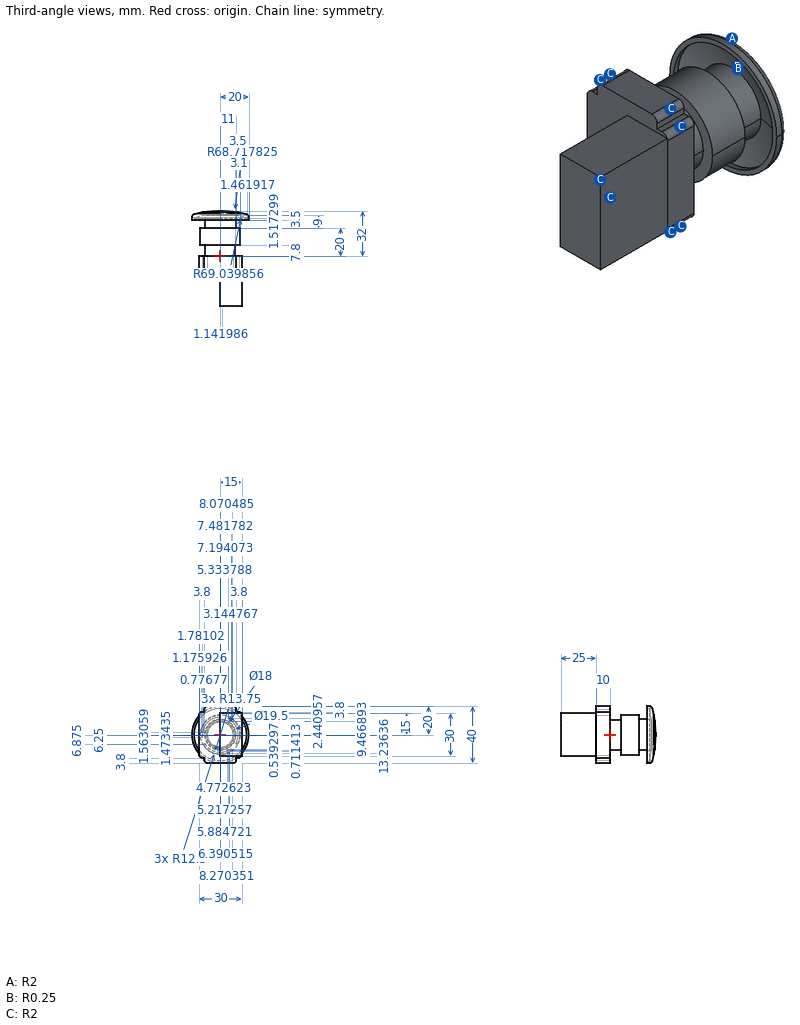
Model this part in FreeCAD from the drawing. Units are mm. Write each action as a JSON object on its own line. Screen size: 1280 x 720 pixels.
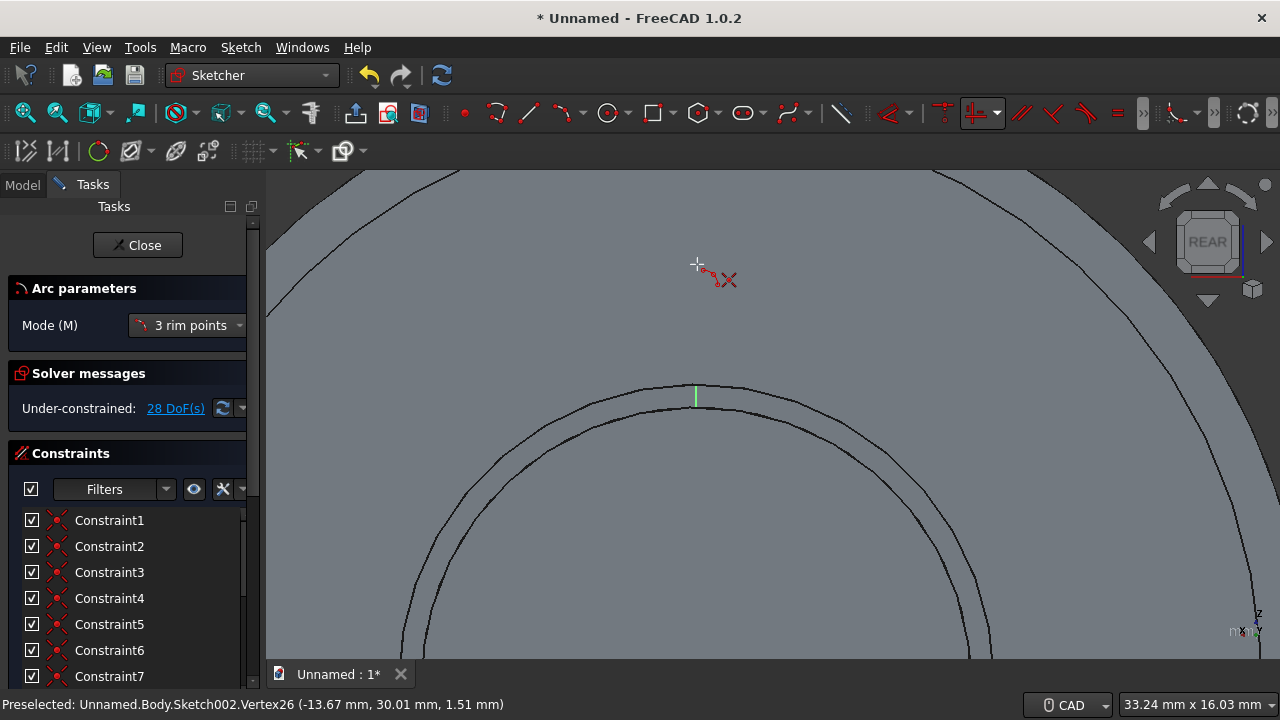
{"action": "left_click", "coordinate": [696, 264]}
{"action": "left_click", "coordinate": [976, 369]}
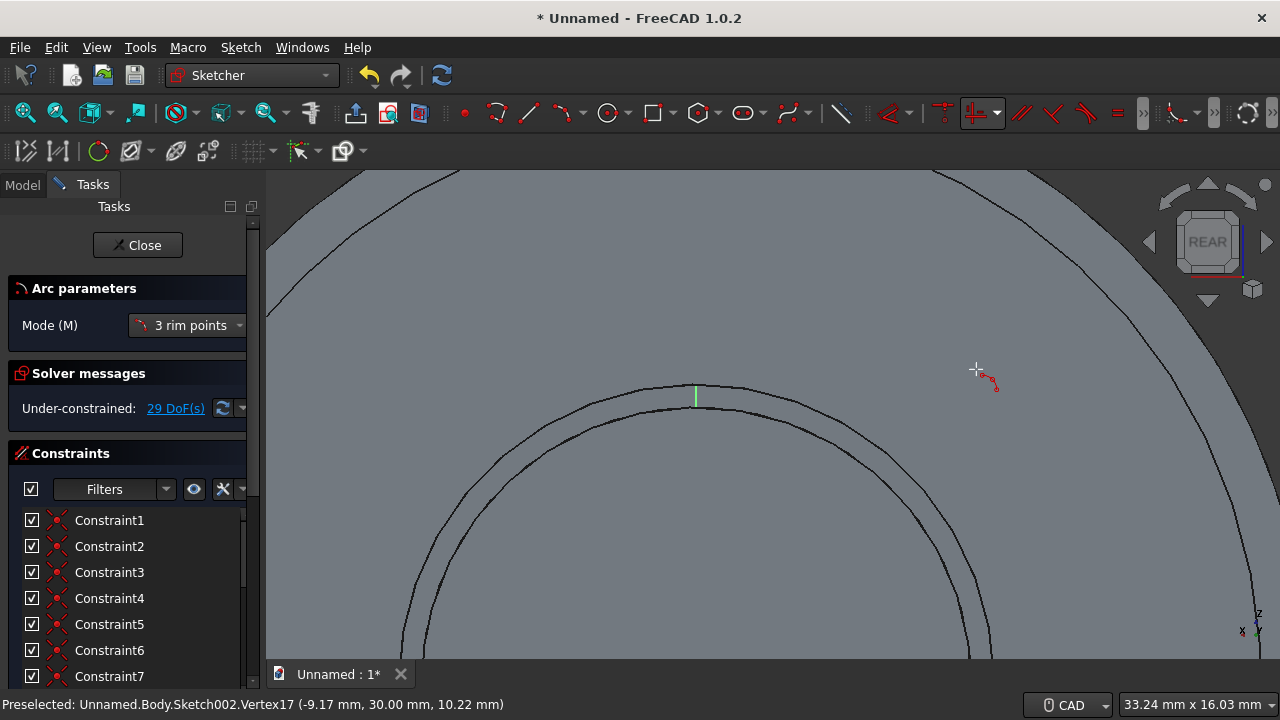
{"action": "left_click", "coordinate": [530, 114]}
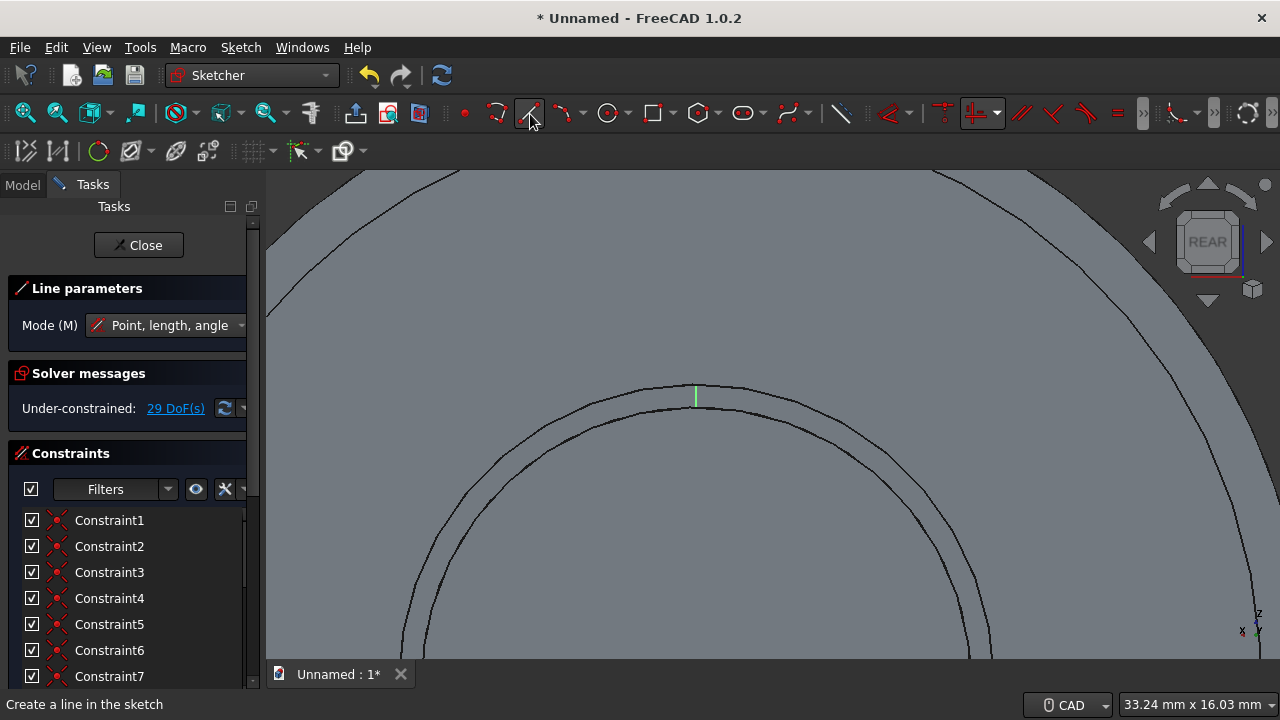
{"action": "scroll", "coordinate": [697, 263], "scroll_direction": "down", "scroll_amount": 5}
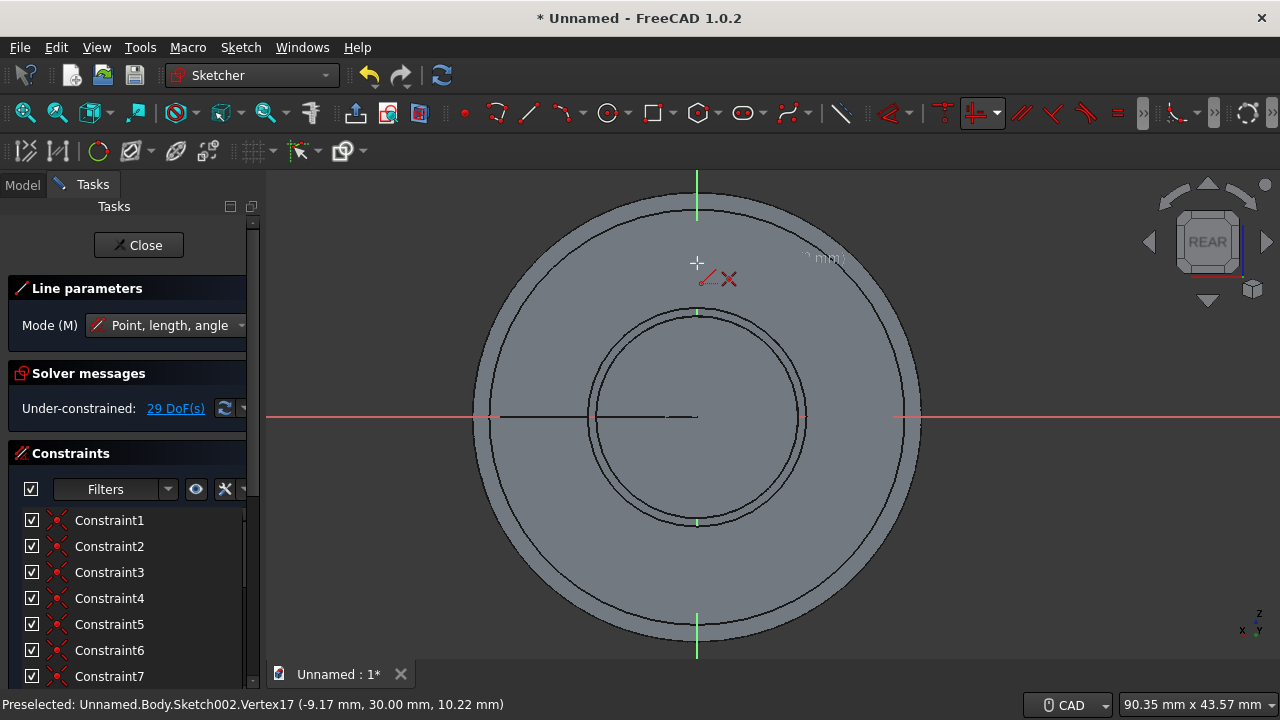
{"action": "left_click", "coordinate": [563, 494]}
{"action": "left_click", "coordinate": [576, 487]}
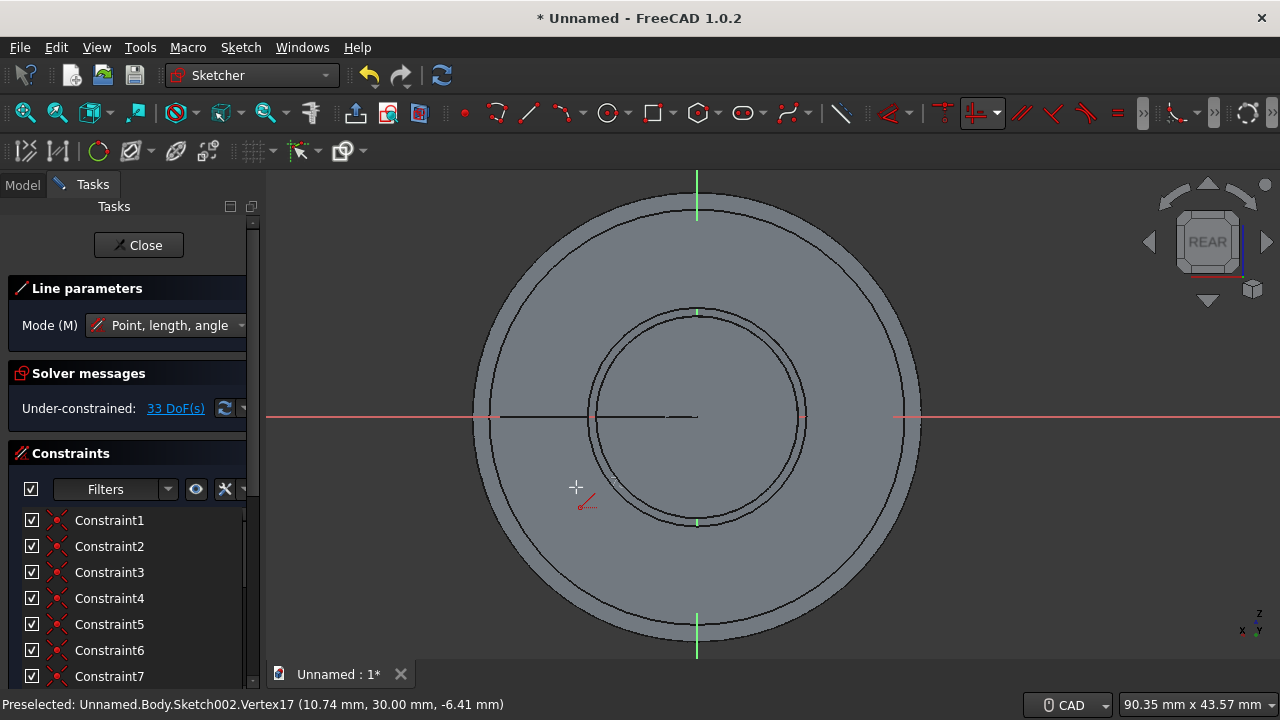
{"action": "left_click", "coordinate": [498, 114]}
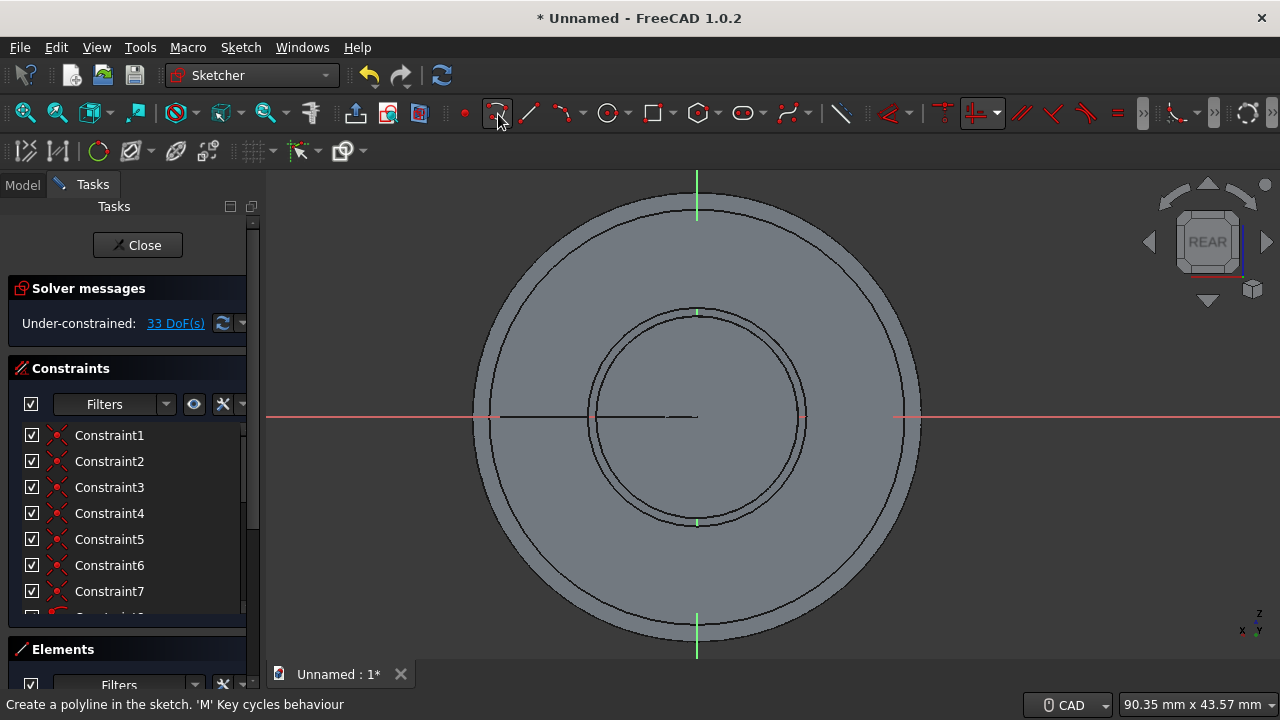
{"action": "left_click", "coordinate": [613, 305]}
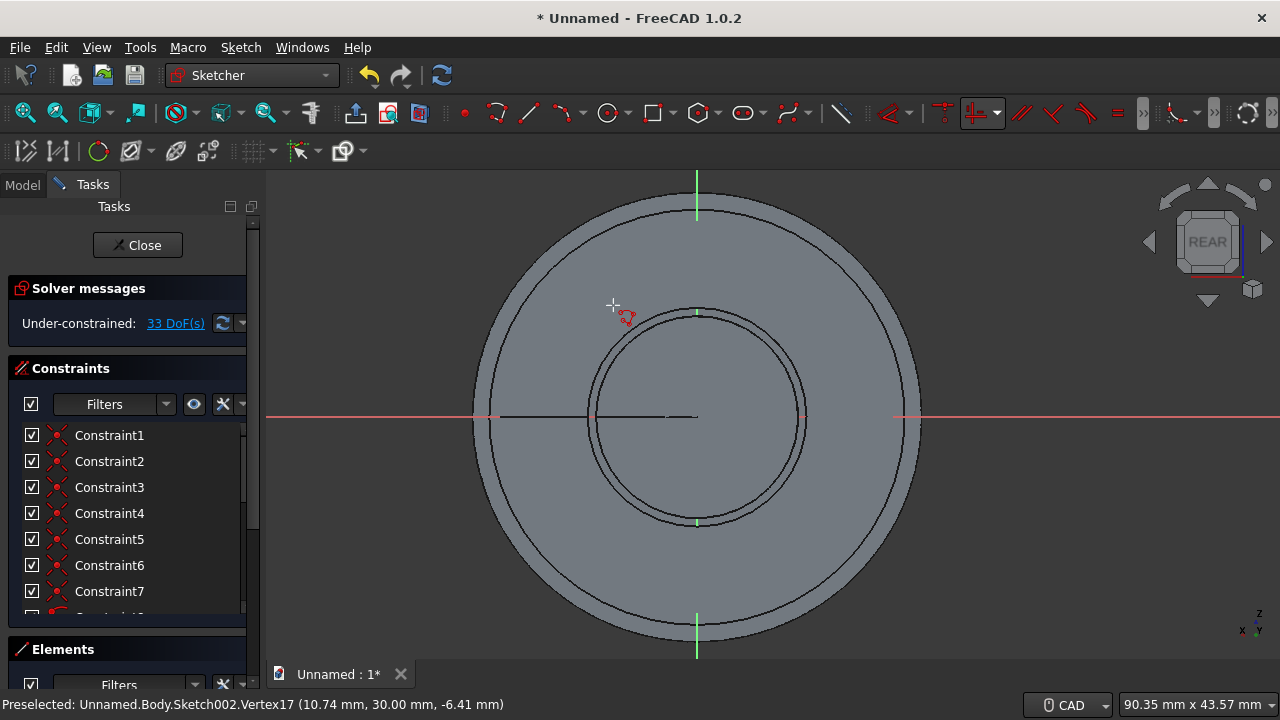
{"action": "scroll", "coordinate": [616, 311], "scroll_direction": "up", "scroll_amount": 5}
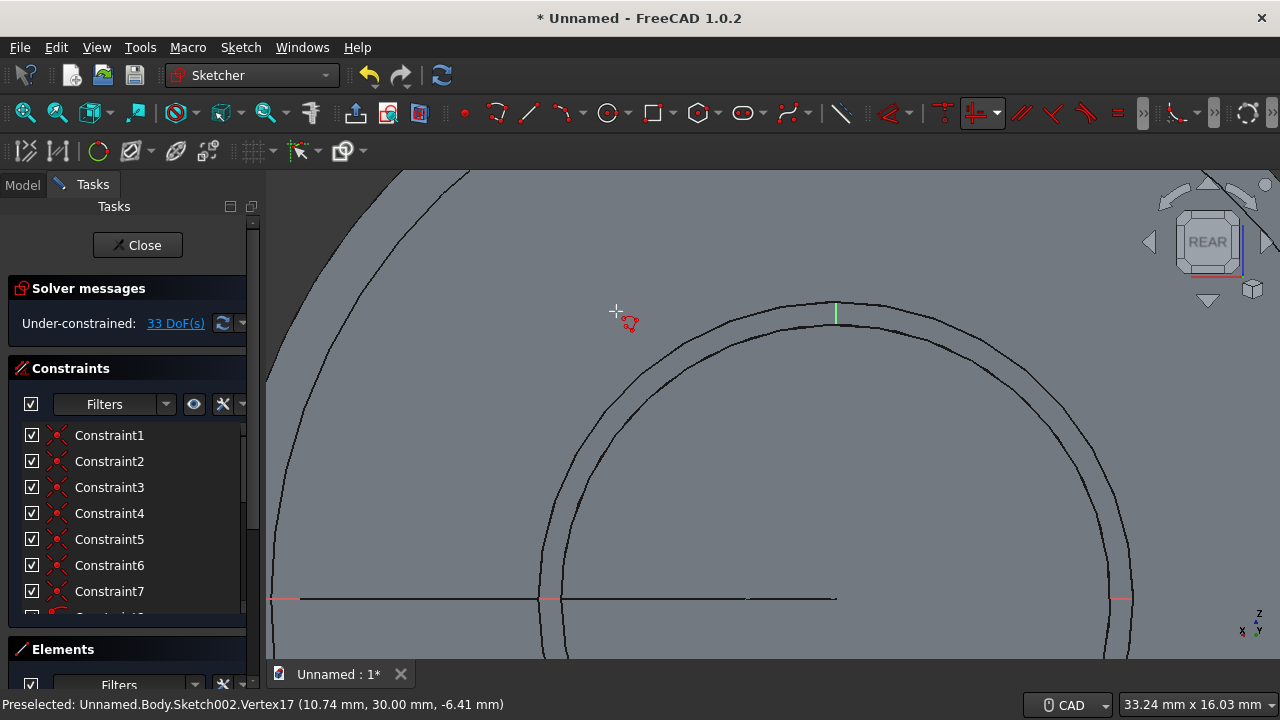
{"action": "left_click", "coordinate": [616, 310]}
{"action": "left_click", "coordinate": [673, 236]}
{"action": "left_click", "coordinate": [577, 236]}
{"action": "left_click", "coordinate": [590, 260]}
{"action": "right_click", "coordinate": [590, 260]}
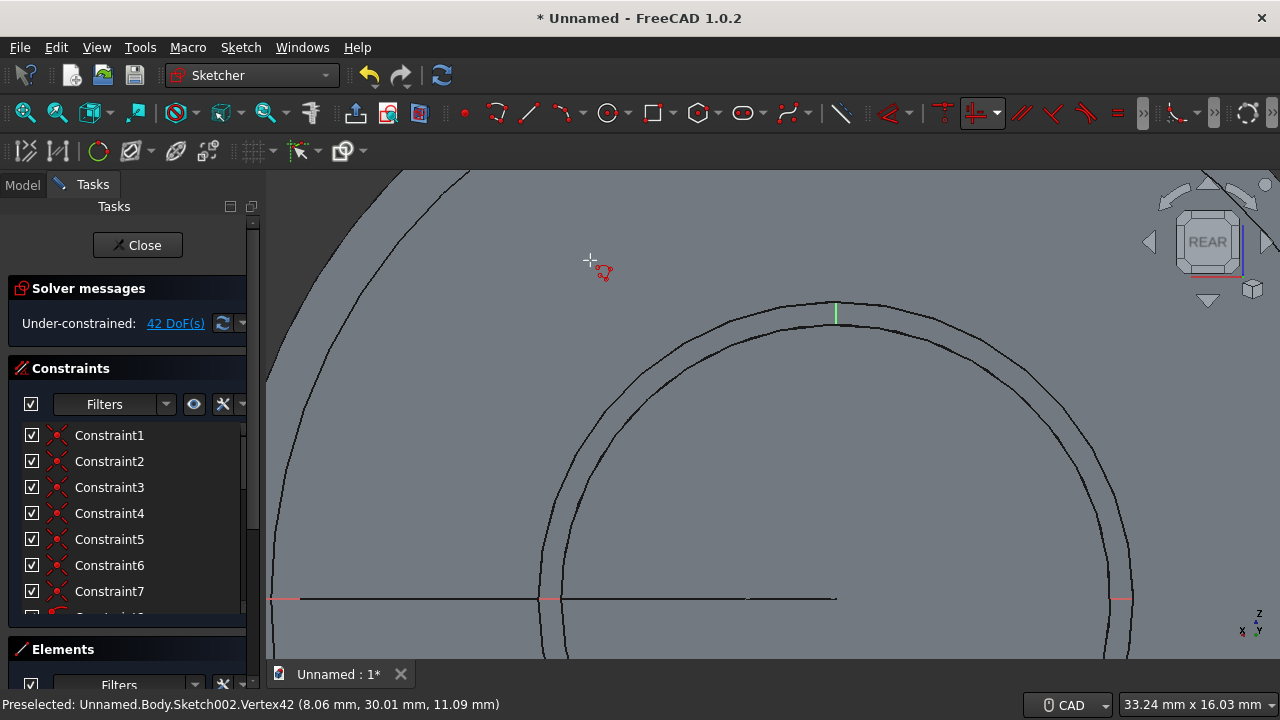
{"action": "left_click", "coordinate": [562, 114]}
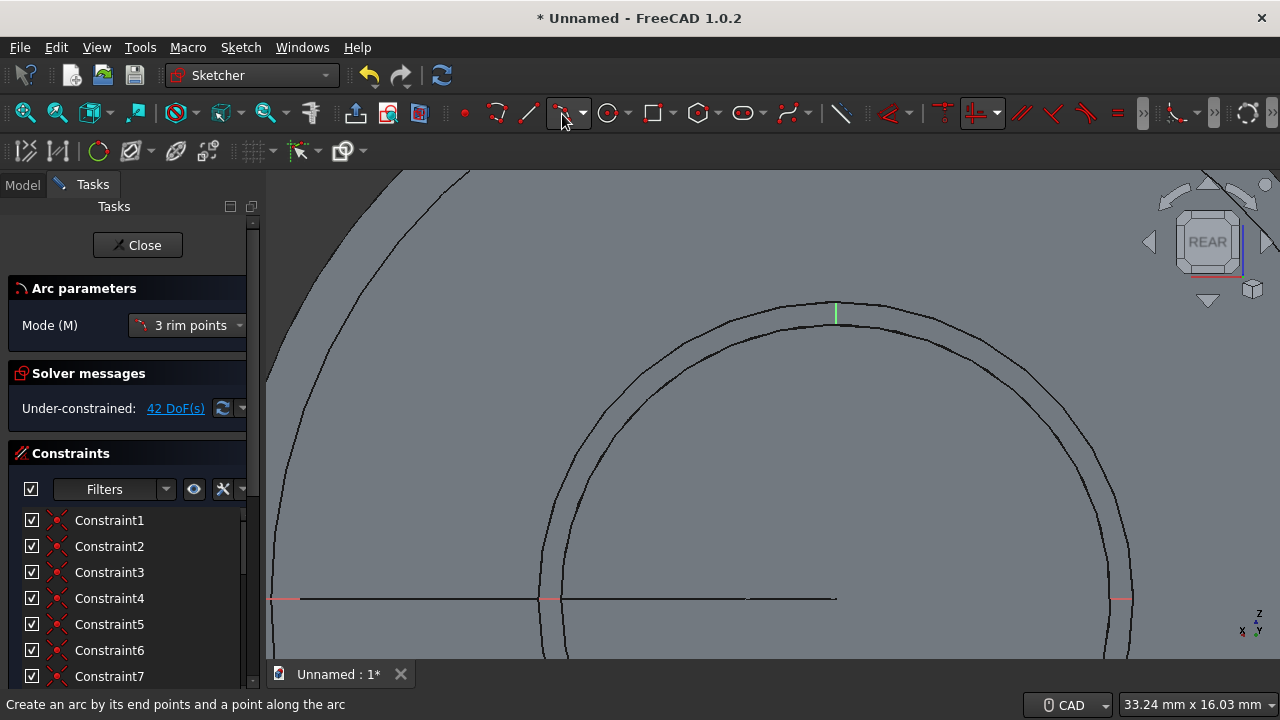
{"action": "scroll", "coordinate": [616, 312], "scroll_direction": "down", "scroll_amount": 5}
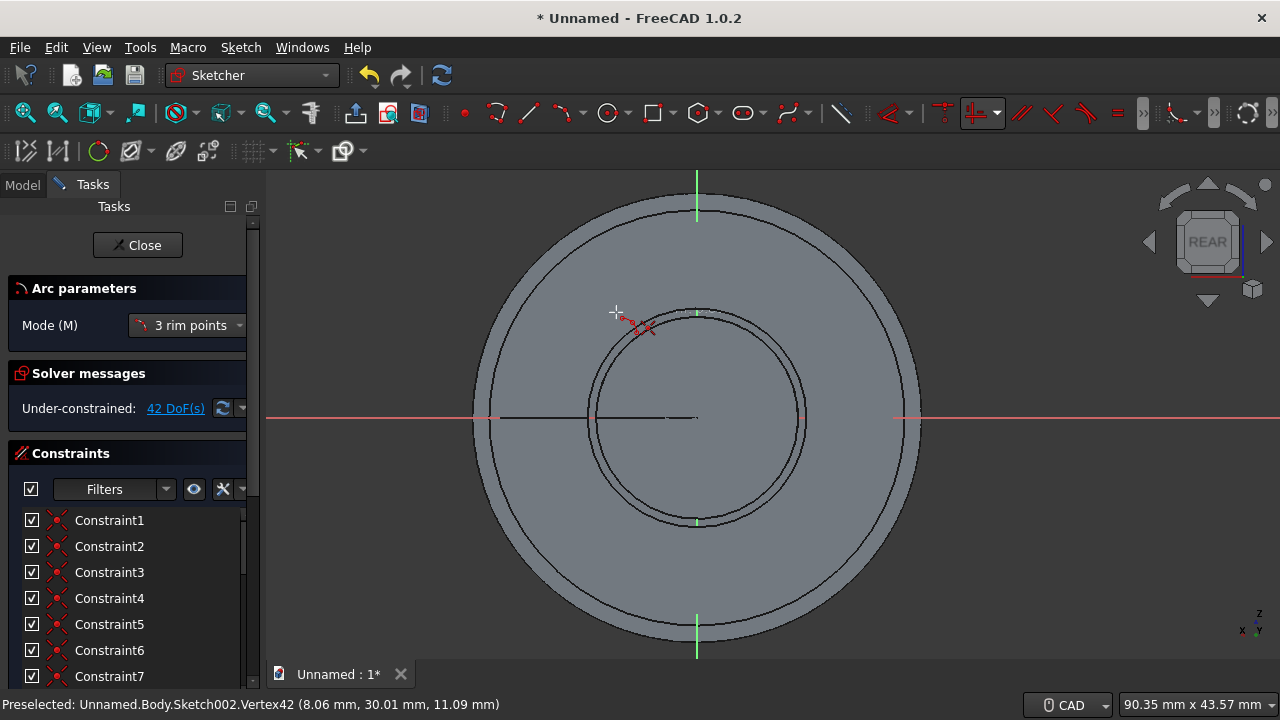
{"action": "scroll", "coordinate": [576, 488], "scroll_direction": "up", "scroll_amount": 5}